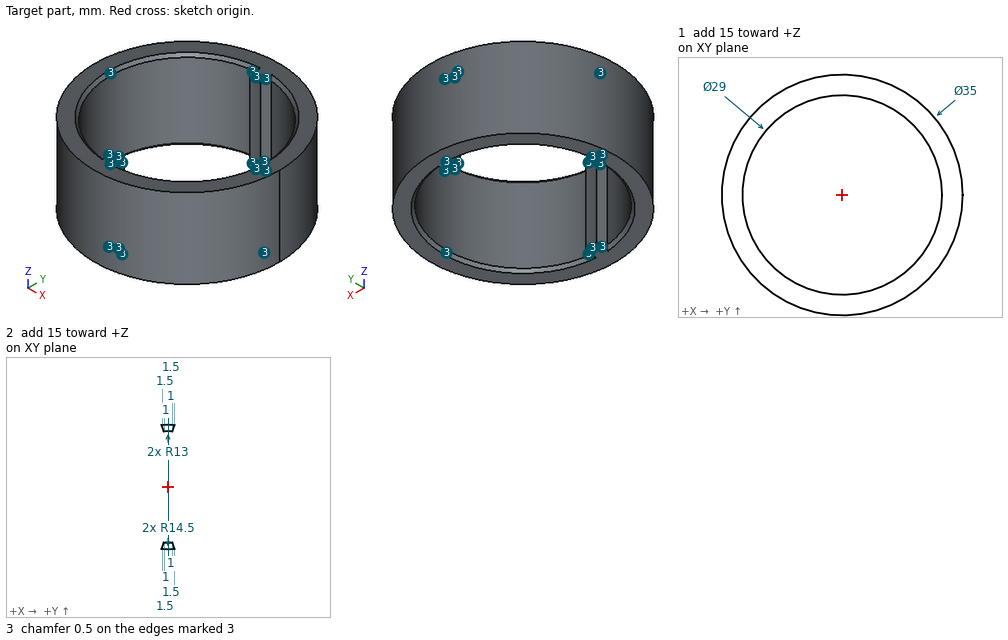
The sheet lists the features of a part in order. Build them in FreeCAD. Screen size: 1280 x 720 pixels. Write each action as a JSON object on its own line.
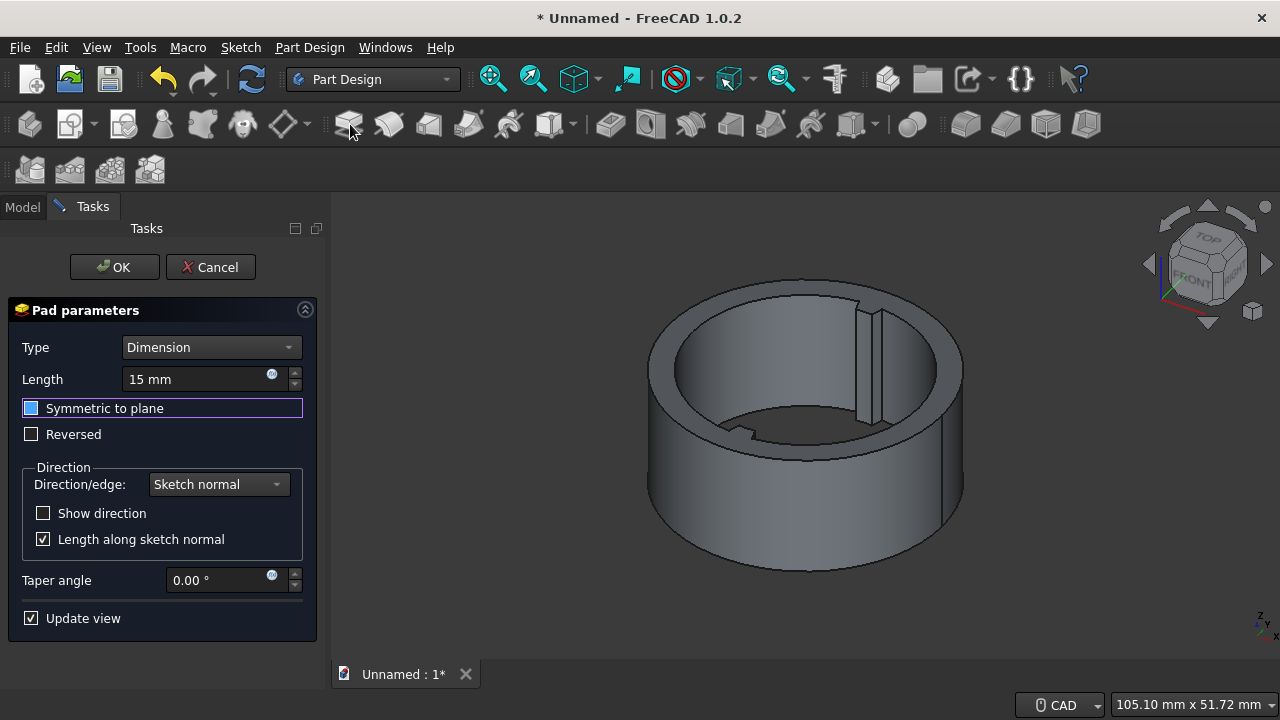
{"action": "left_click", "coordinate": [115, 267]}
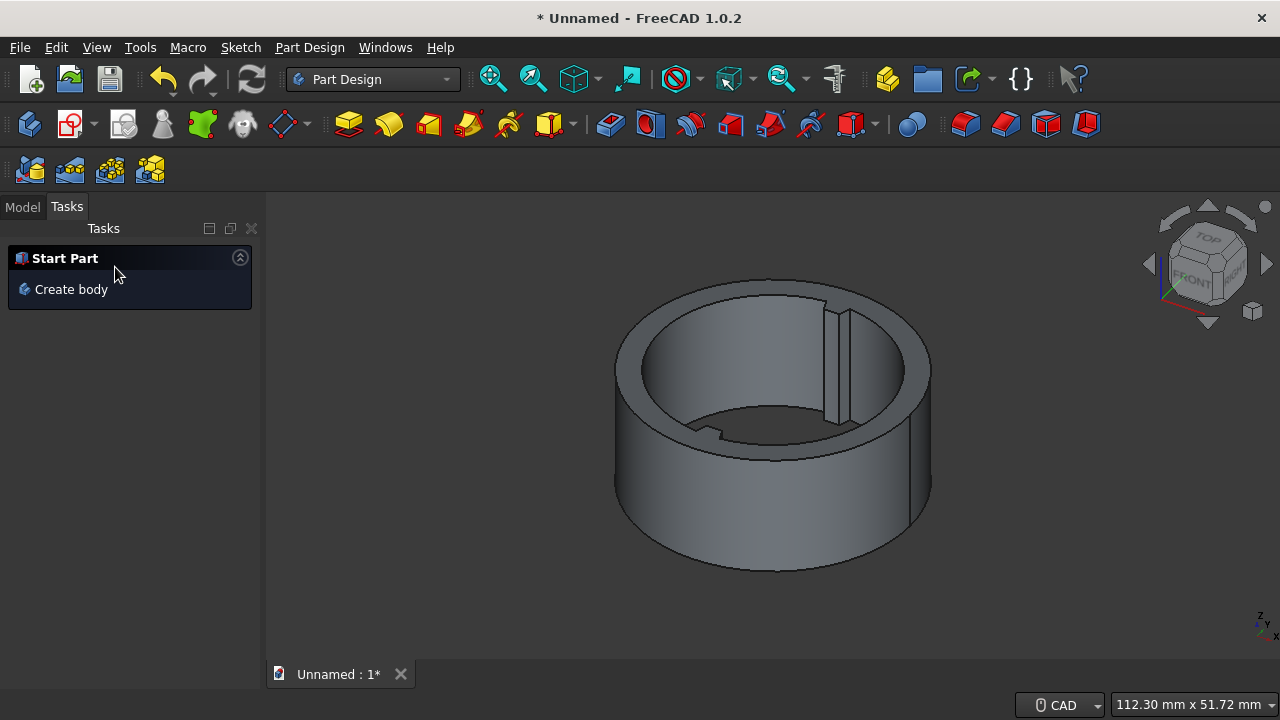
{"action": "left_click", "coordinate": [660, 331]}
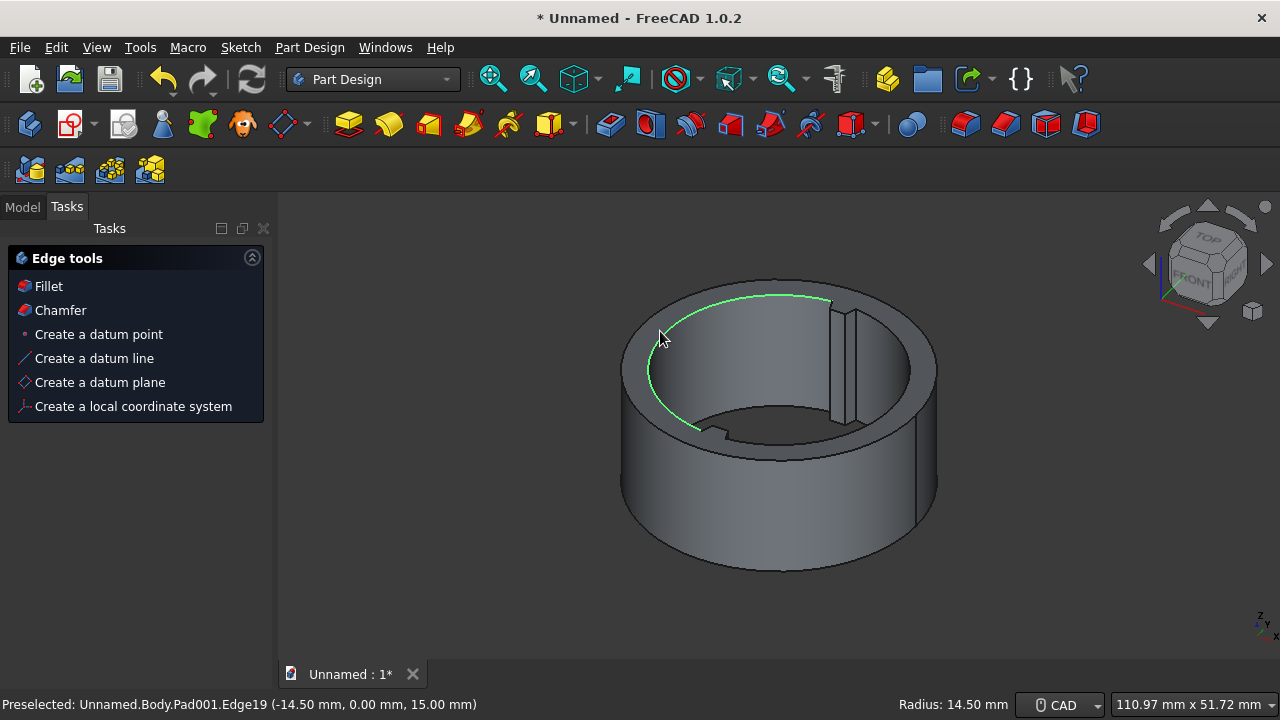
{"action": "left_click", "coordinate": [832, 420], "text": "ctrl"}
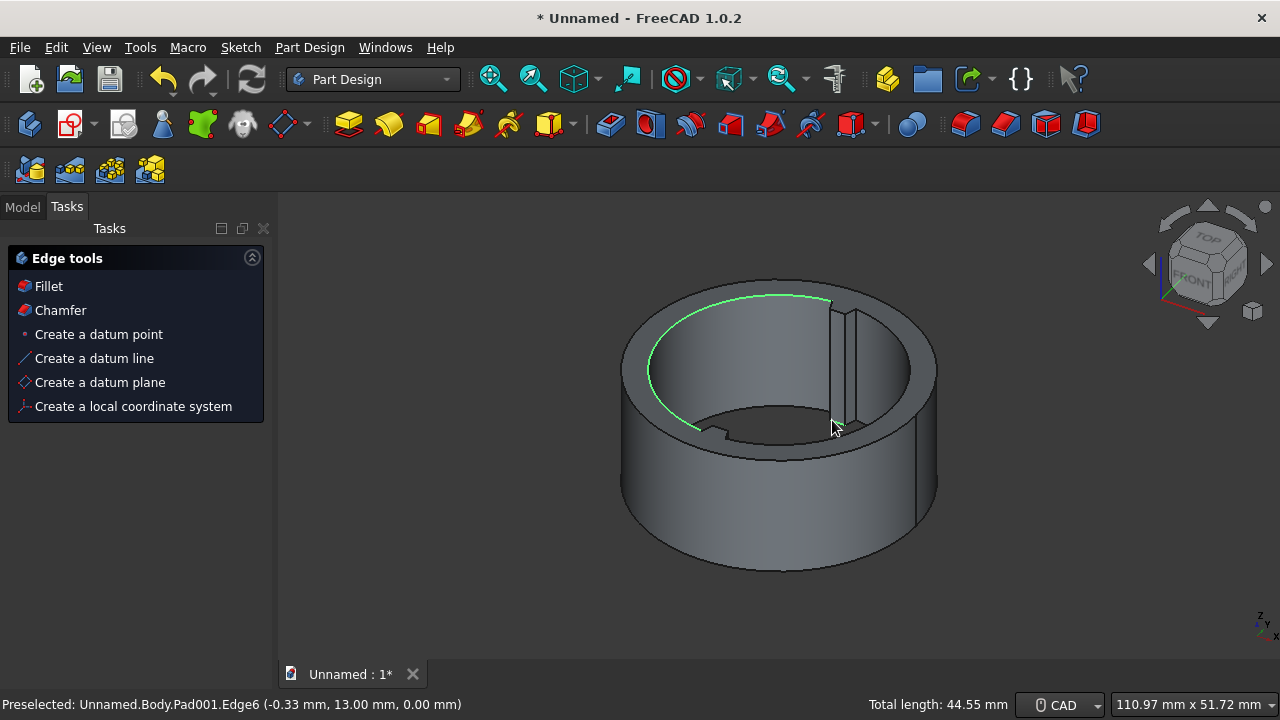
{"action": "left_click", "coordinate": [852, 310], "text": "ctrl"}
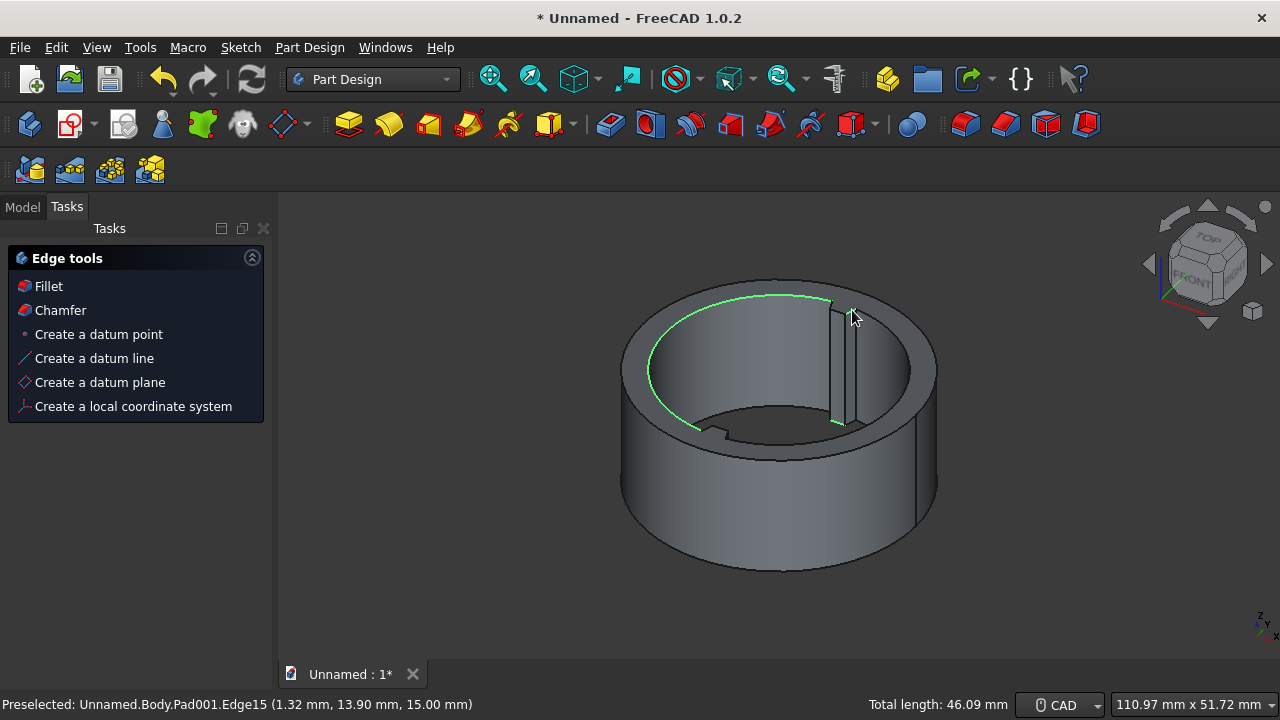
{"action": "left_click", "coordinate": [838, 311], "text": "ctrl"}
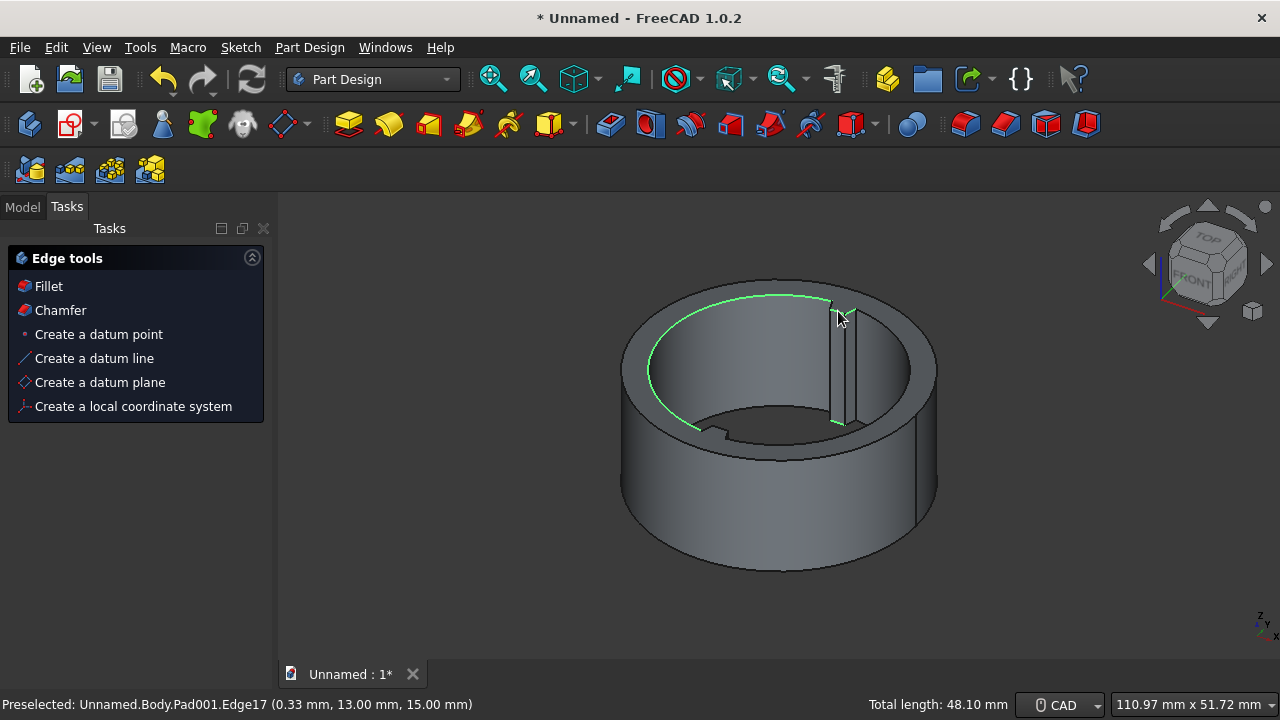
{"action": "left_click", "coordinate": [907, 353], "text": "ctrl"}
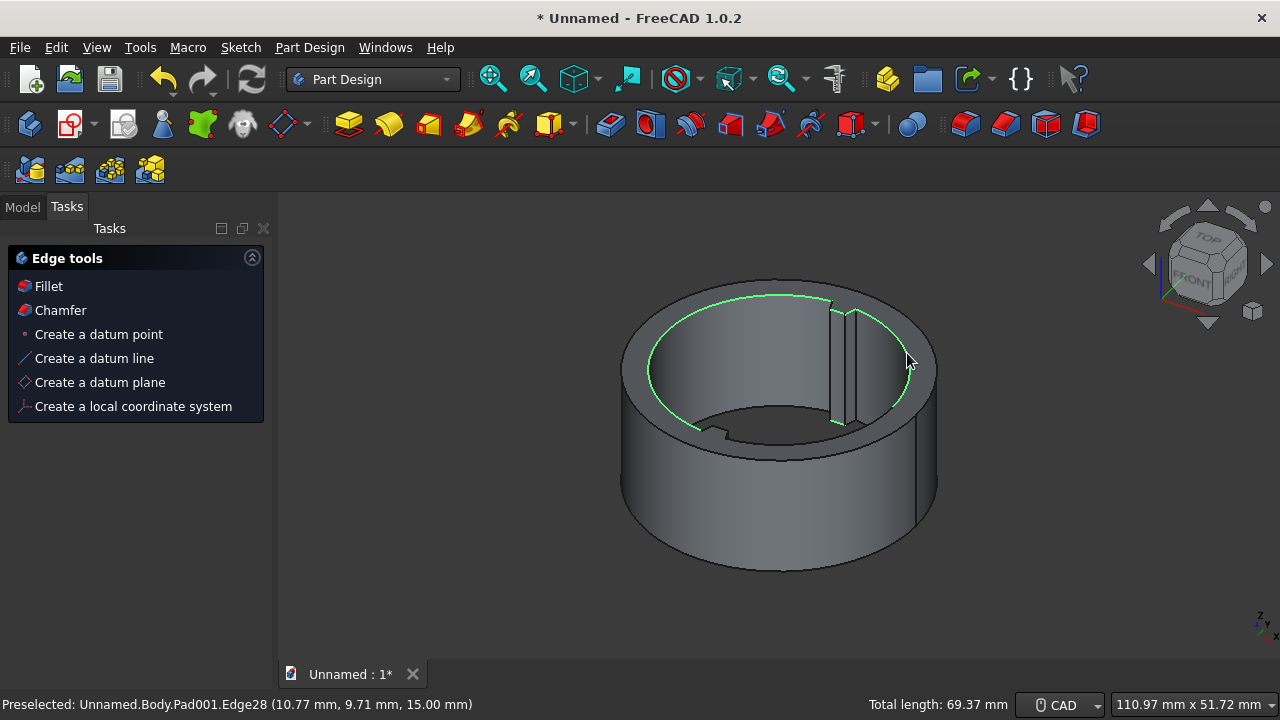
{"action": "left_click", "coordinate": [720, 427], "text": "ctrl"}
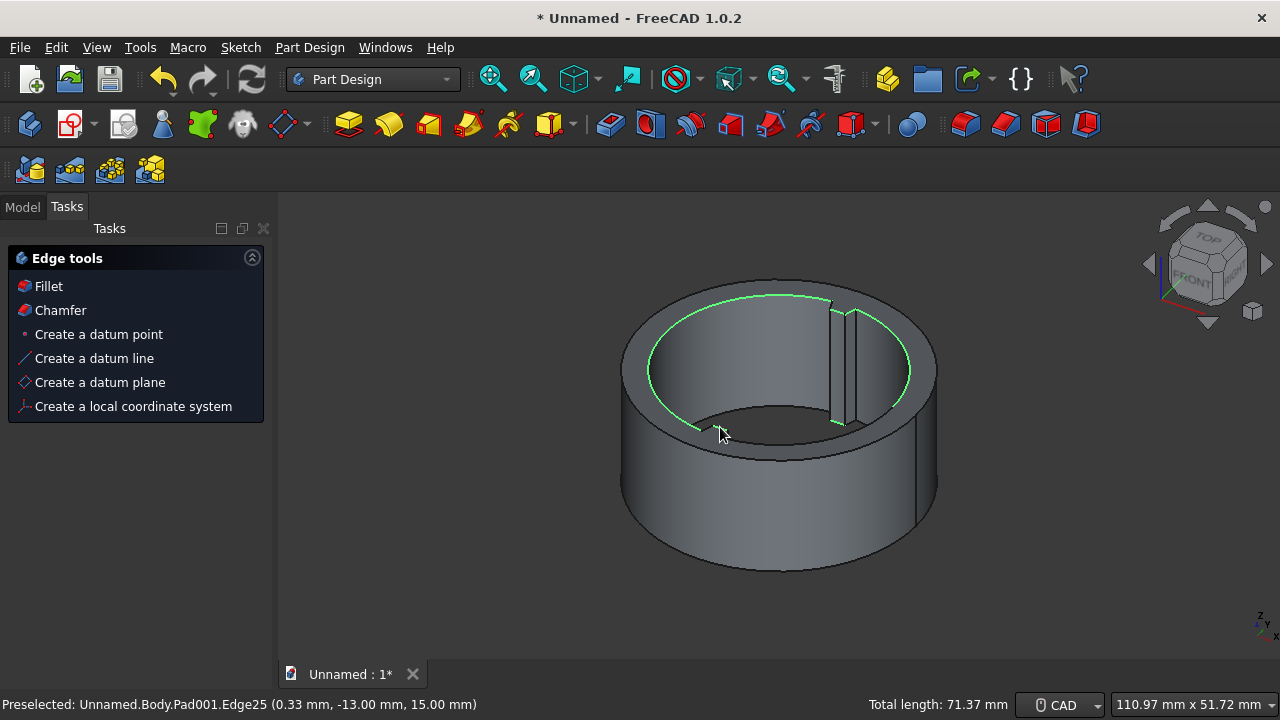
{"action": "key", "text": "0"}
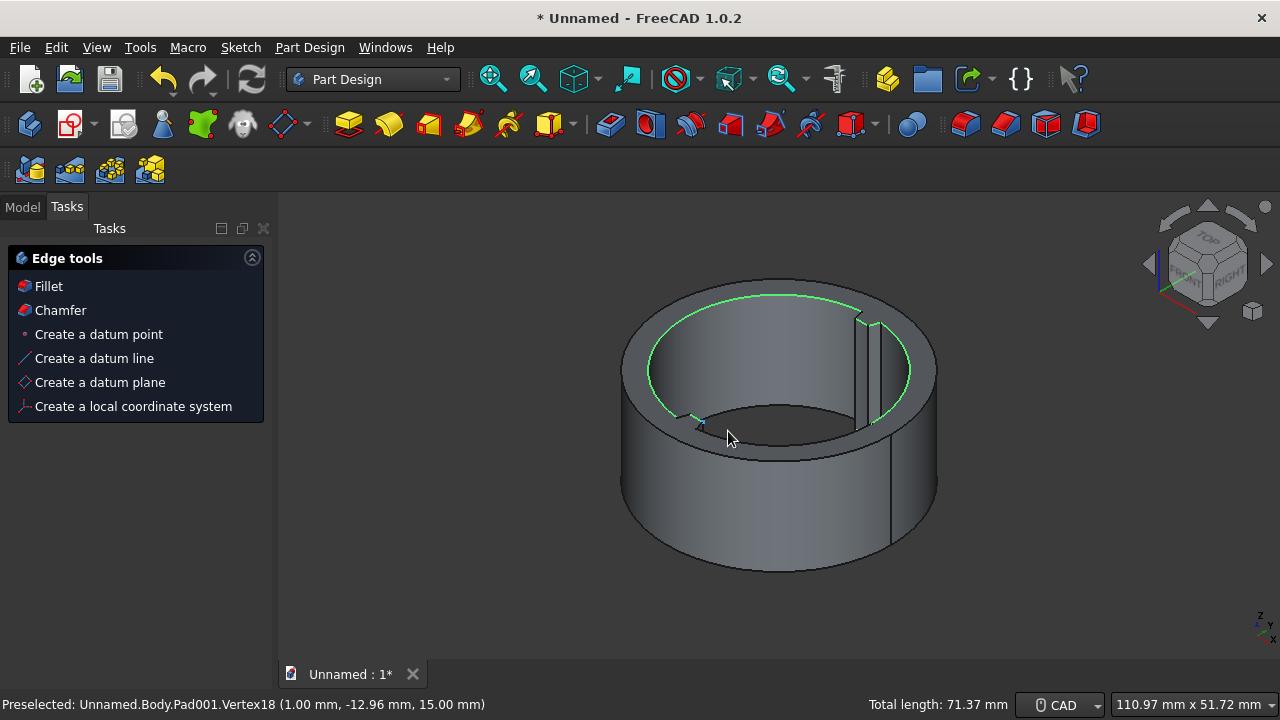
{"action": "key", "text": "2"}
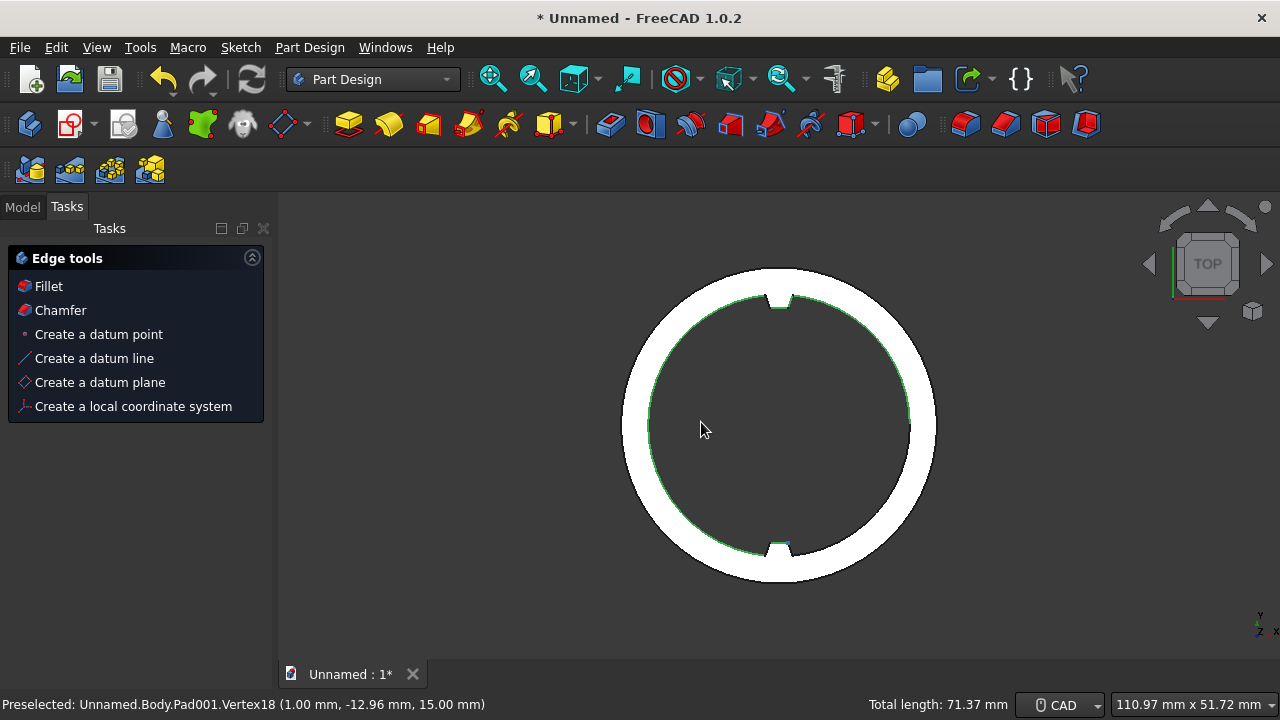
{"action": "left_click", "coordinate": [768, 301], "text": "ctrl"}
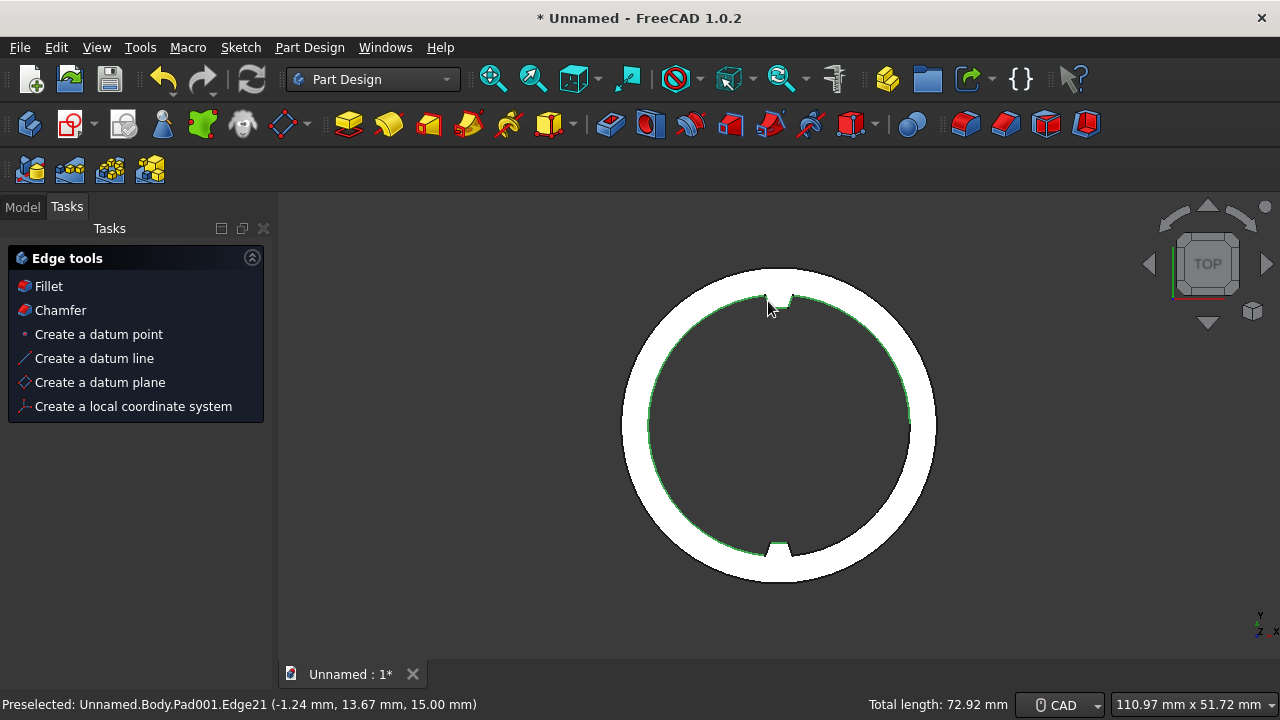
{"action": "left_click", "coordinate": [768, 548], "text": "ctrl"}